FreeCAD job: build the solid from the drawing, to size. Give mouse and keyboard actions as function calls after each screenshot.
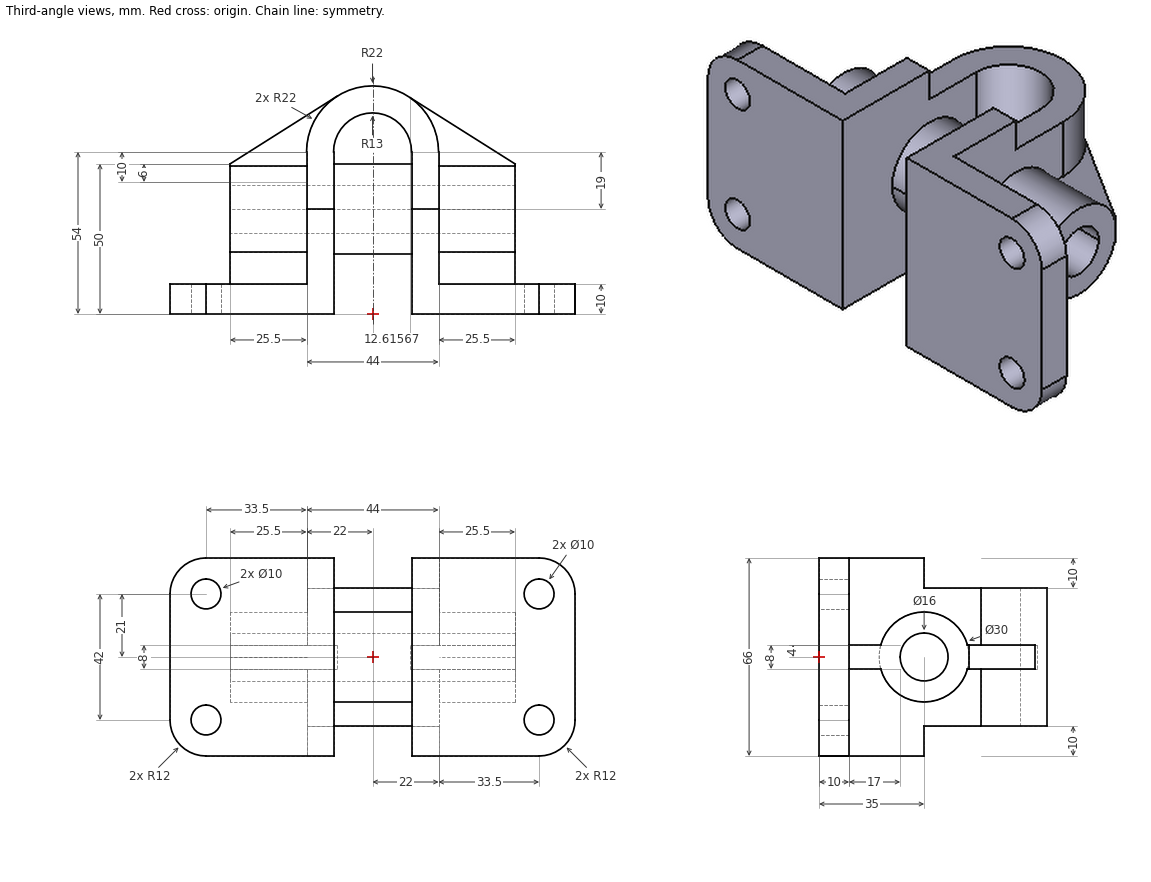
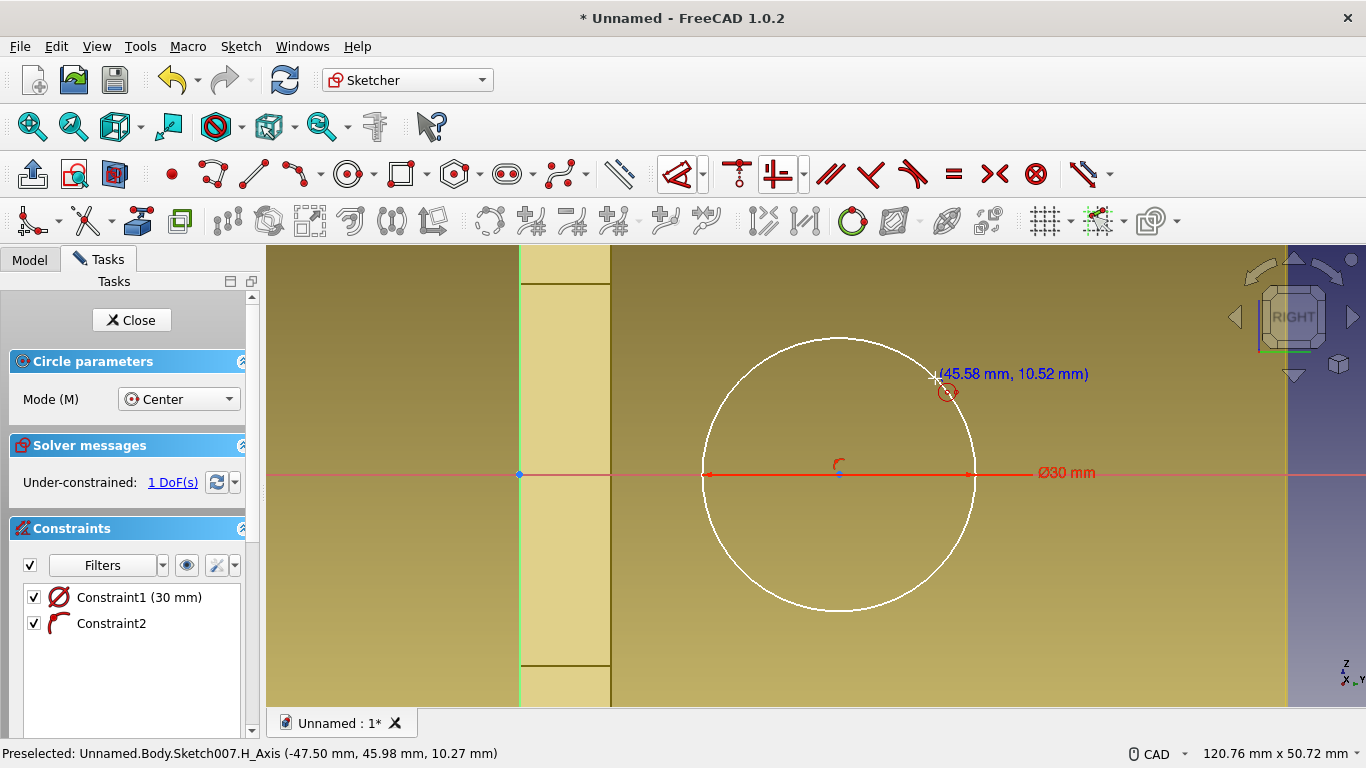
click(839, 475)
move(890, 423)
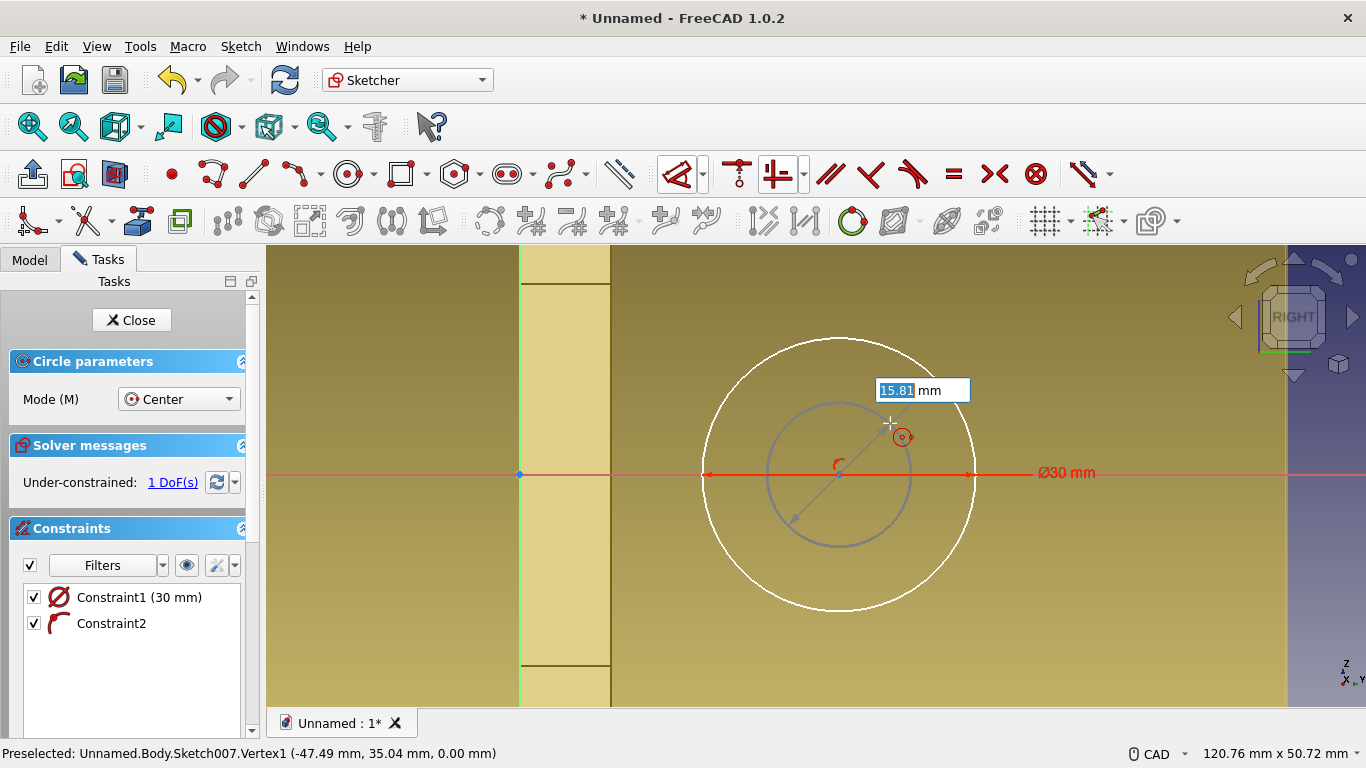
text(16)
key(Return)
key(Escape)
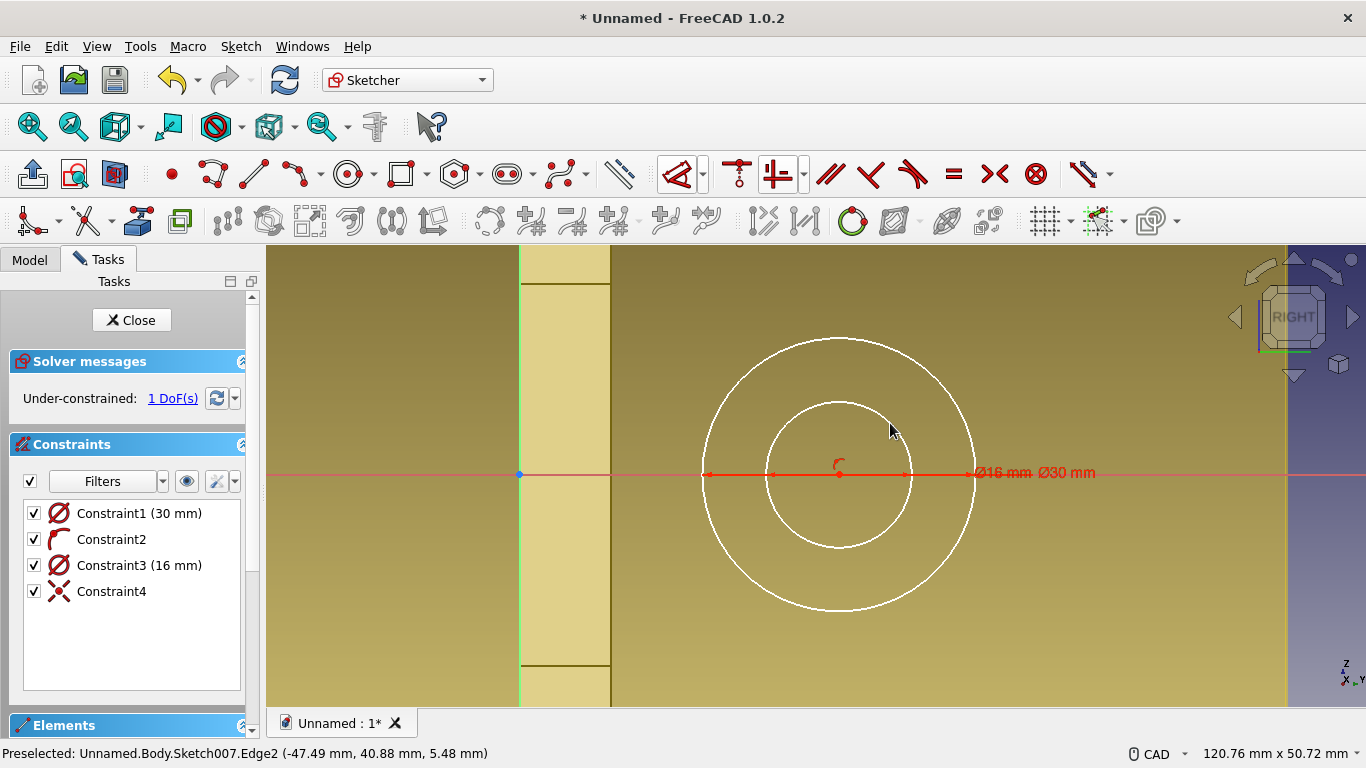
click(839, 475)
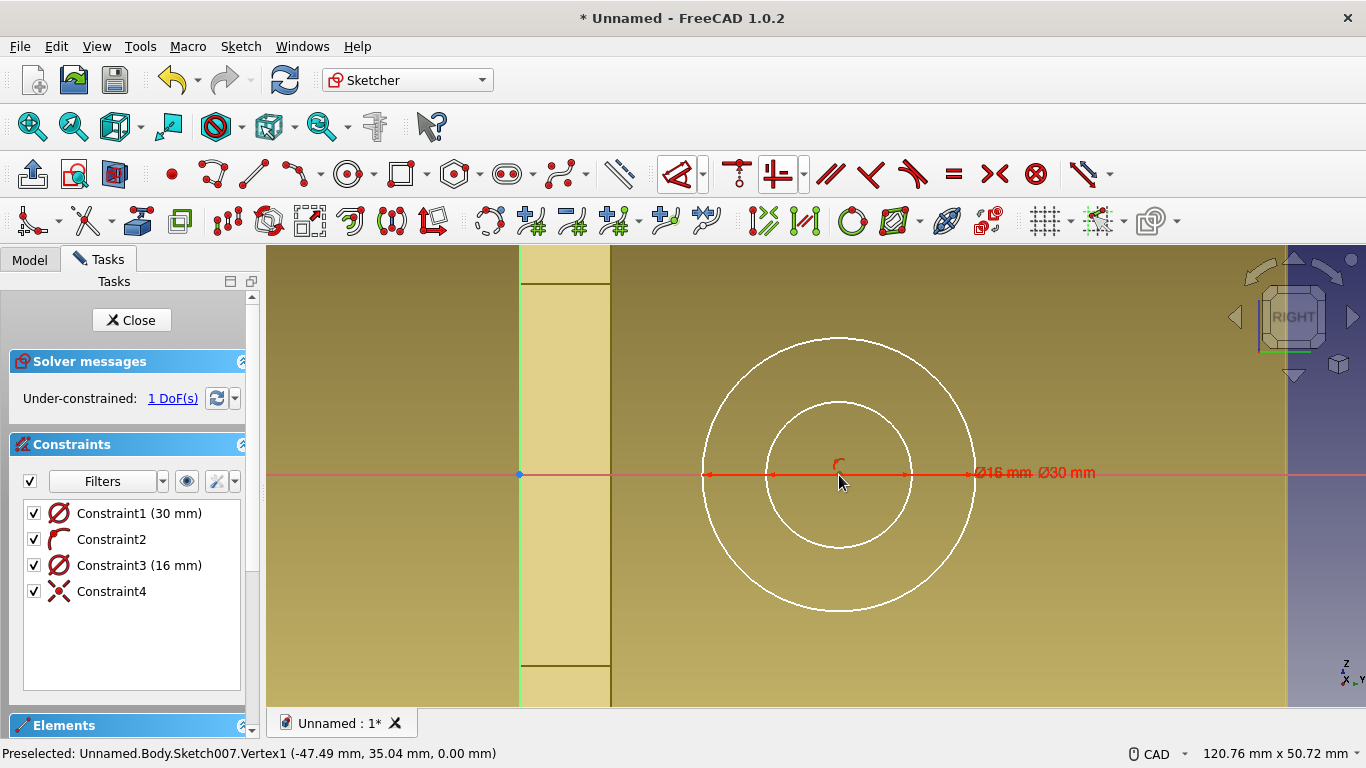
click(702, 174)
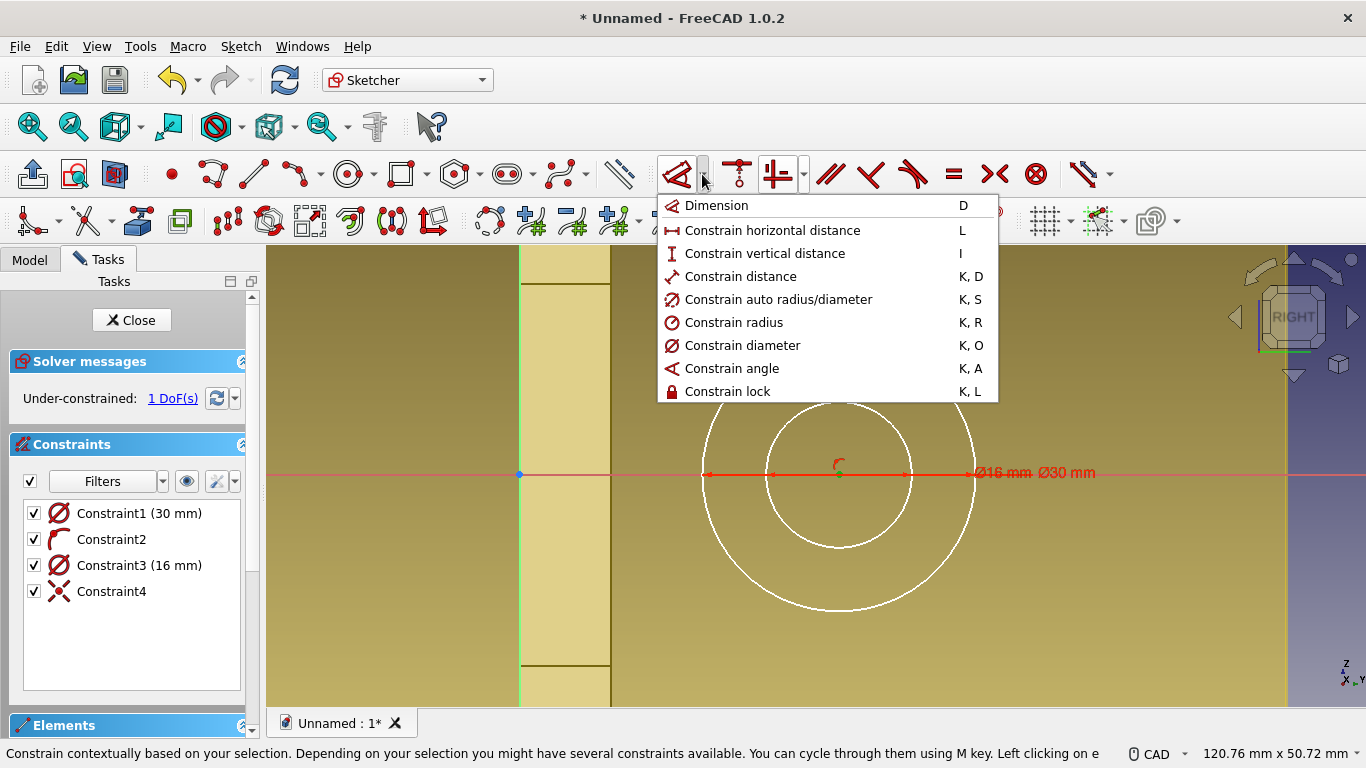
click(828, 230)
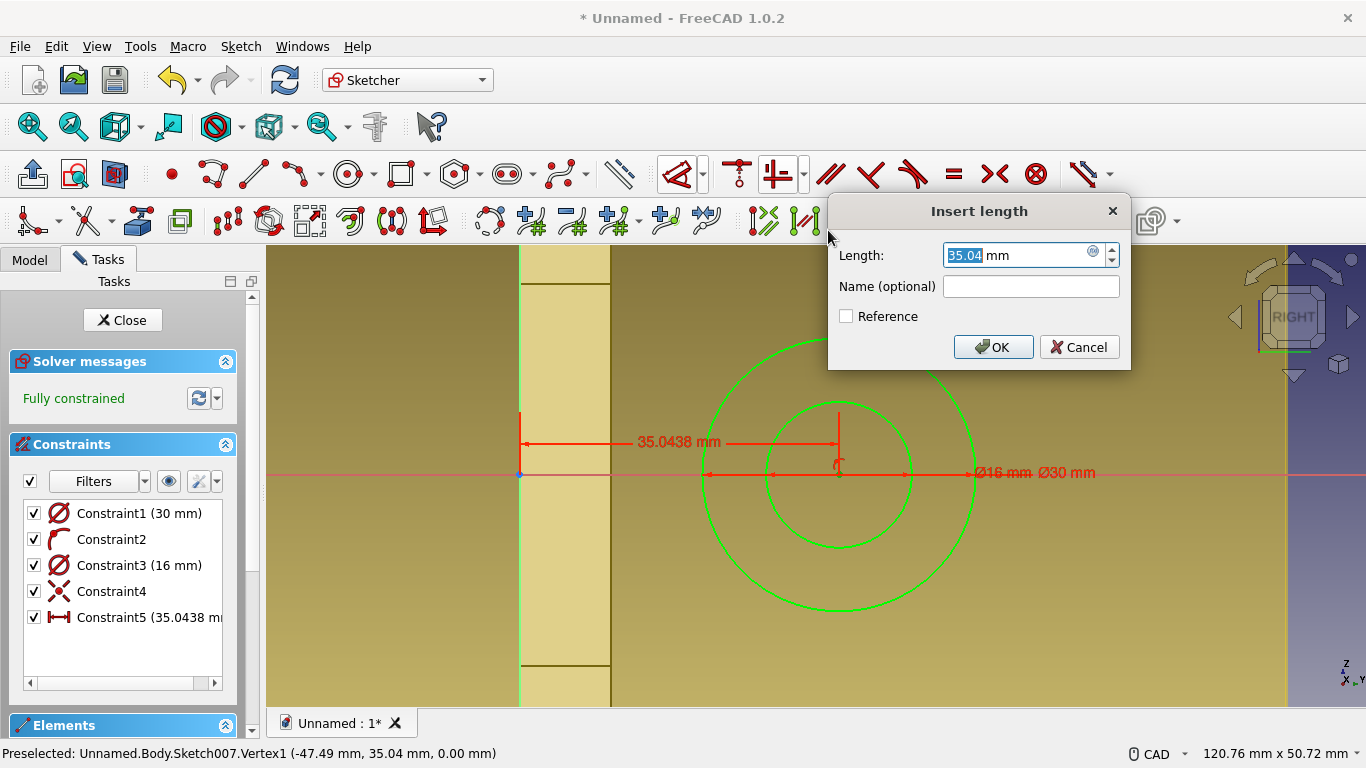
text(35)
key(Return)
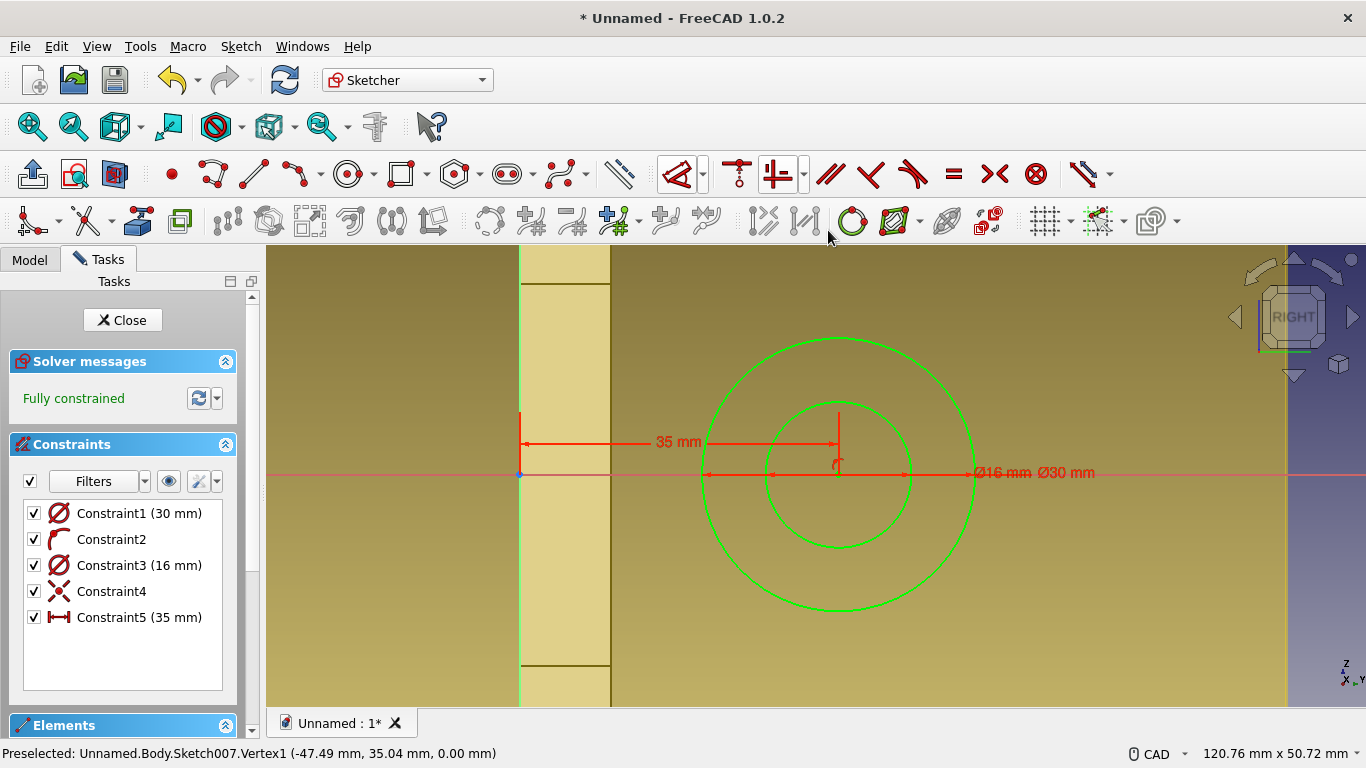
click(123, 320)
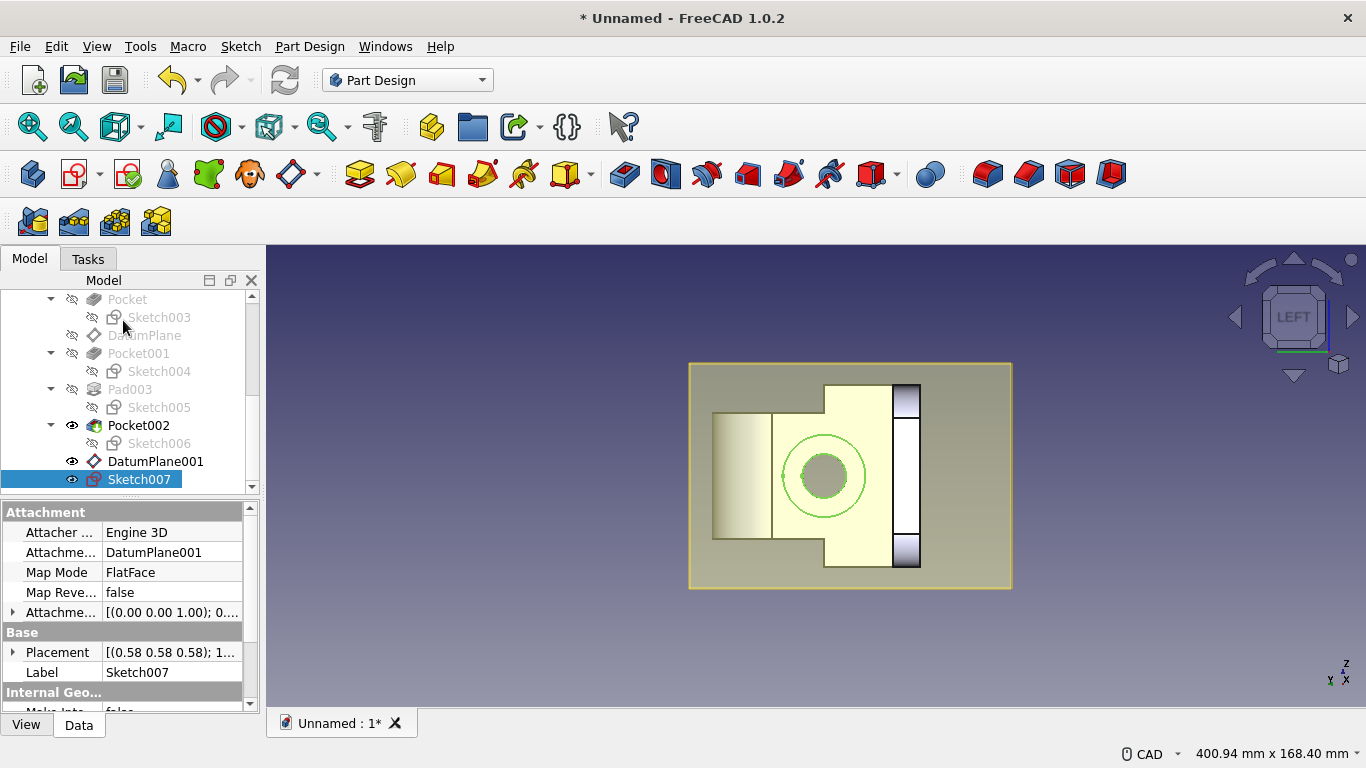
click(360, 174)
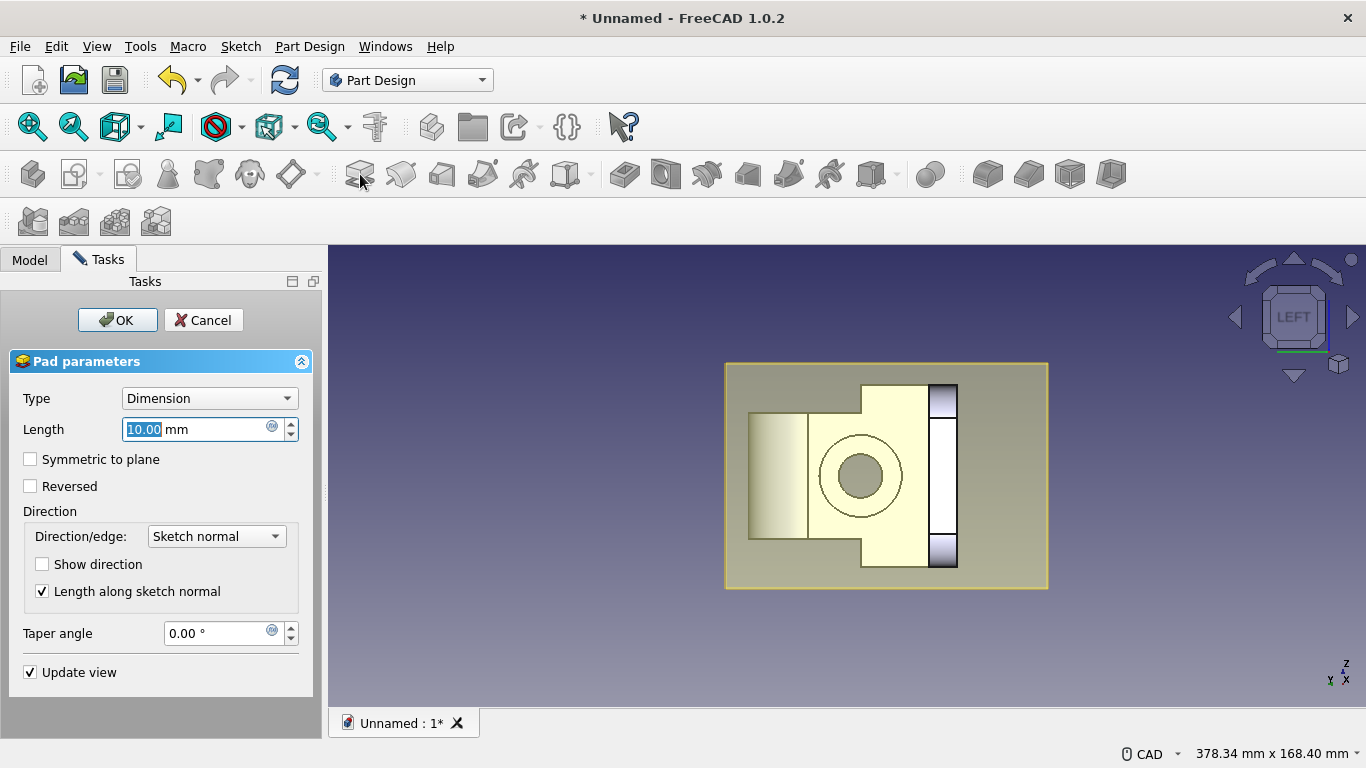
text(25.5)
key(Tab)